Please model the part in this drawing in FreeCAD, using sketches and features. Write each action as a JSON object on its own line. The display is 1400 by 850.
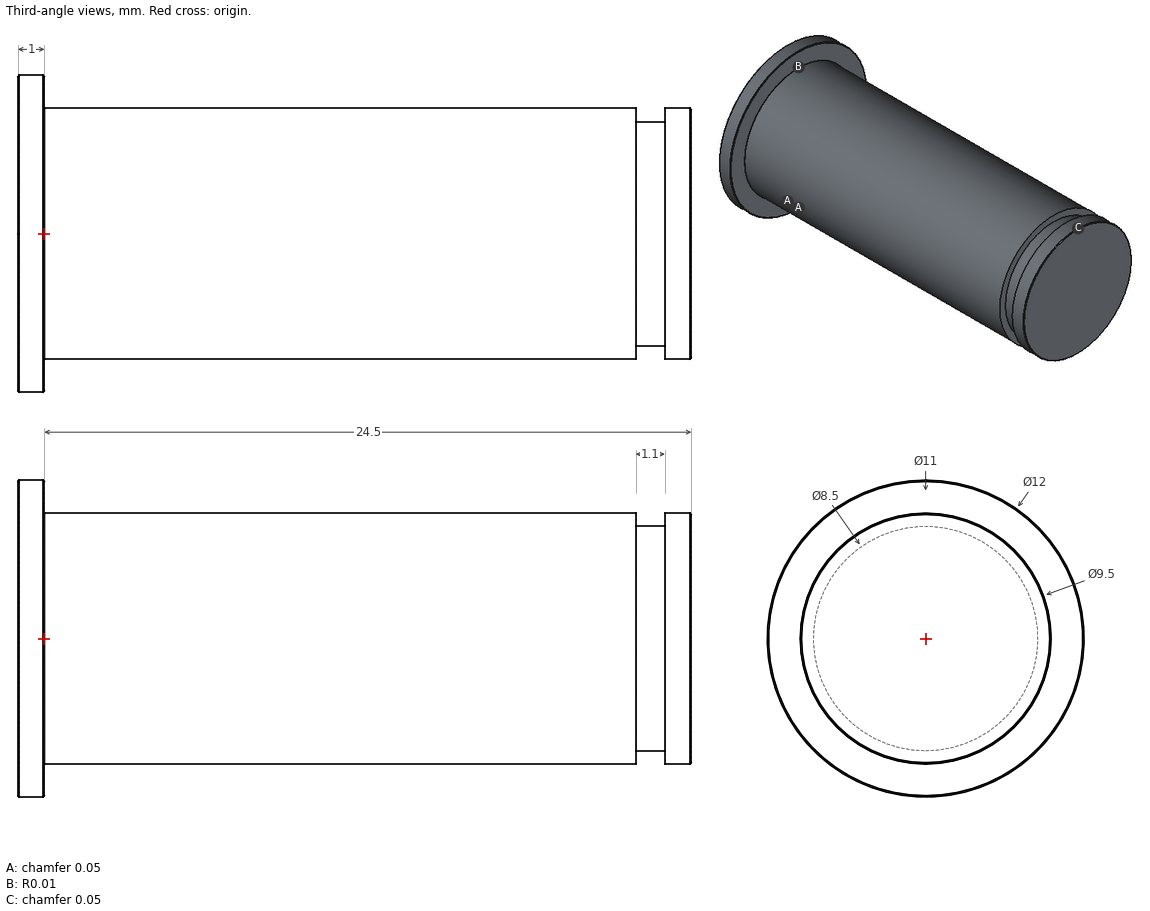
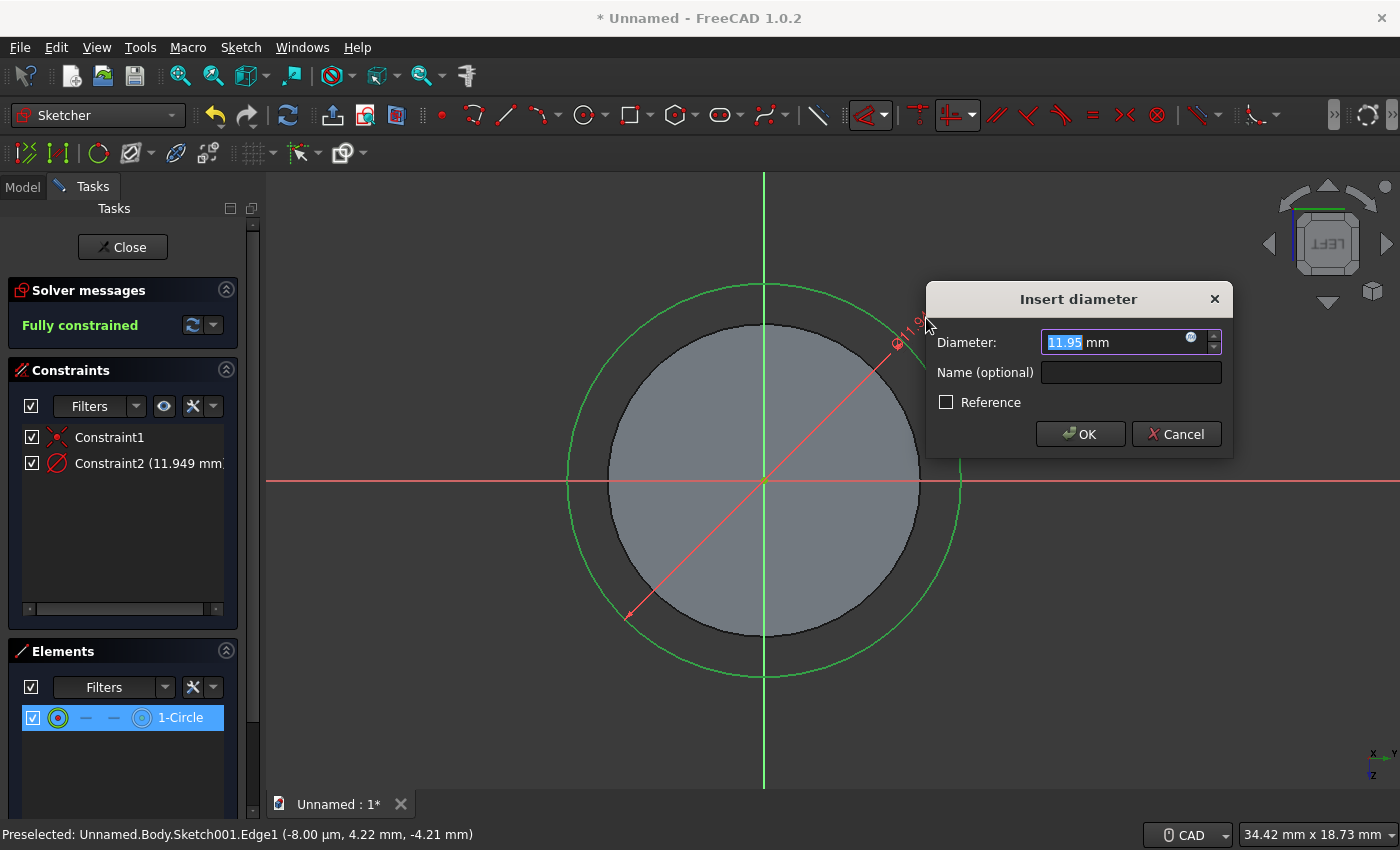
{"action": "type", "text": "12"}
{"action": "key", "text": "Return"}
{"action": "key", "text": "Escape"}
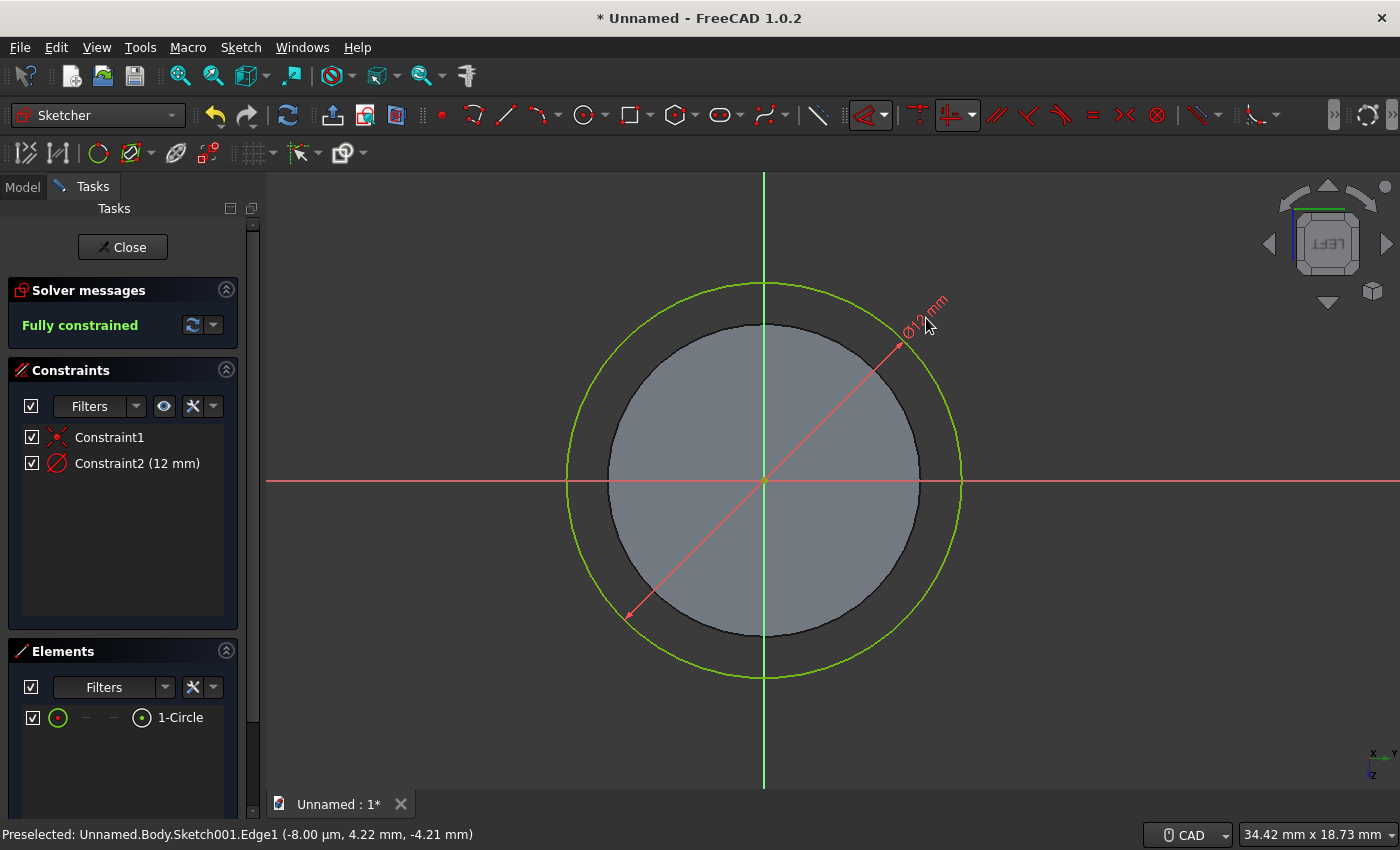
{"action": "left_click", "coordinate": [123, 247]}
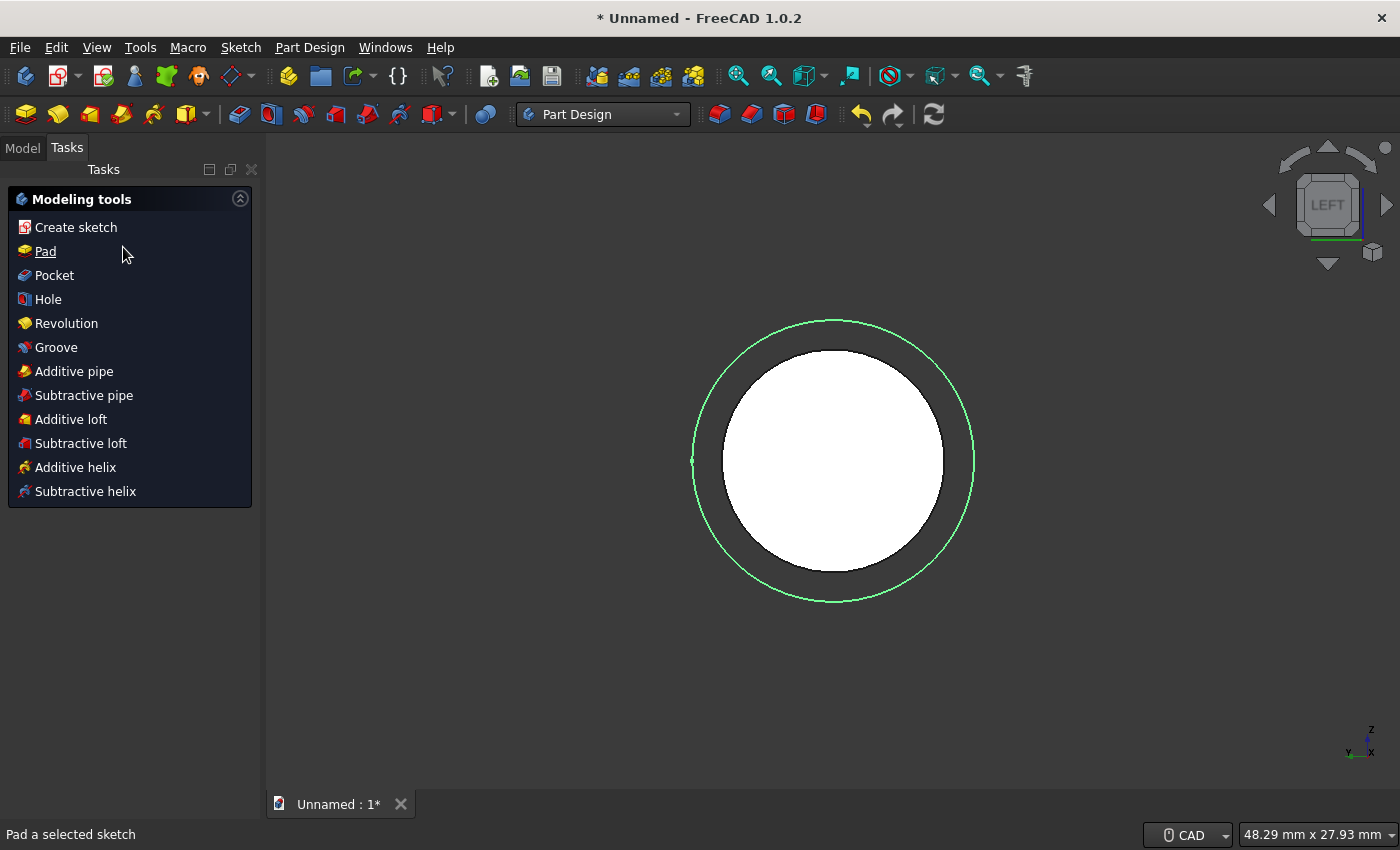
{"action": "left_click", "coordinate": [26, 114]}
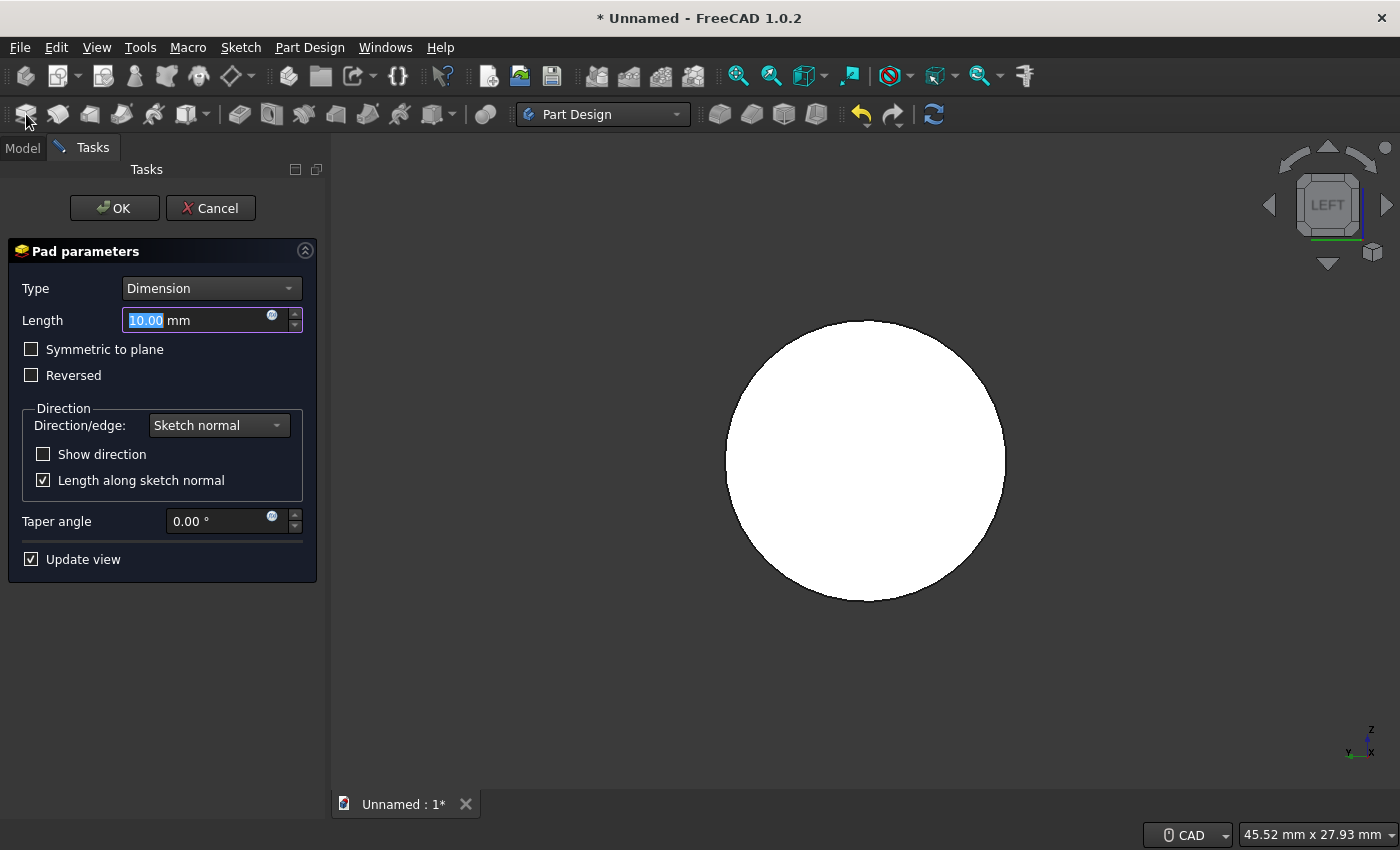
{"action": "type", "text": "1"}
{"action": "key", "text": "Tab"}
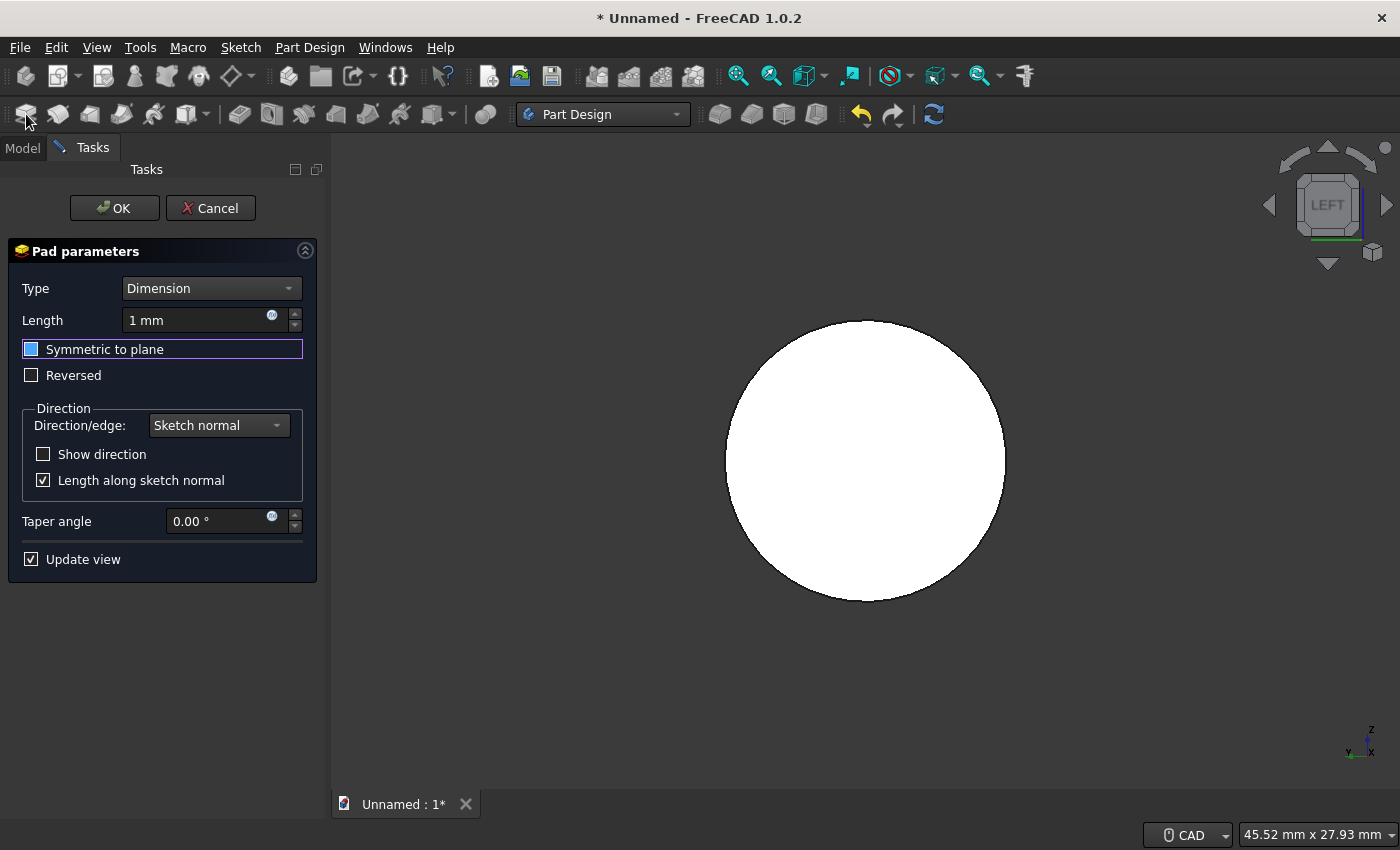
{"action": "left_click", "coordinate": [115, 208]}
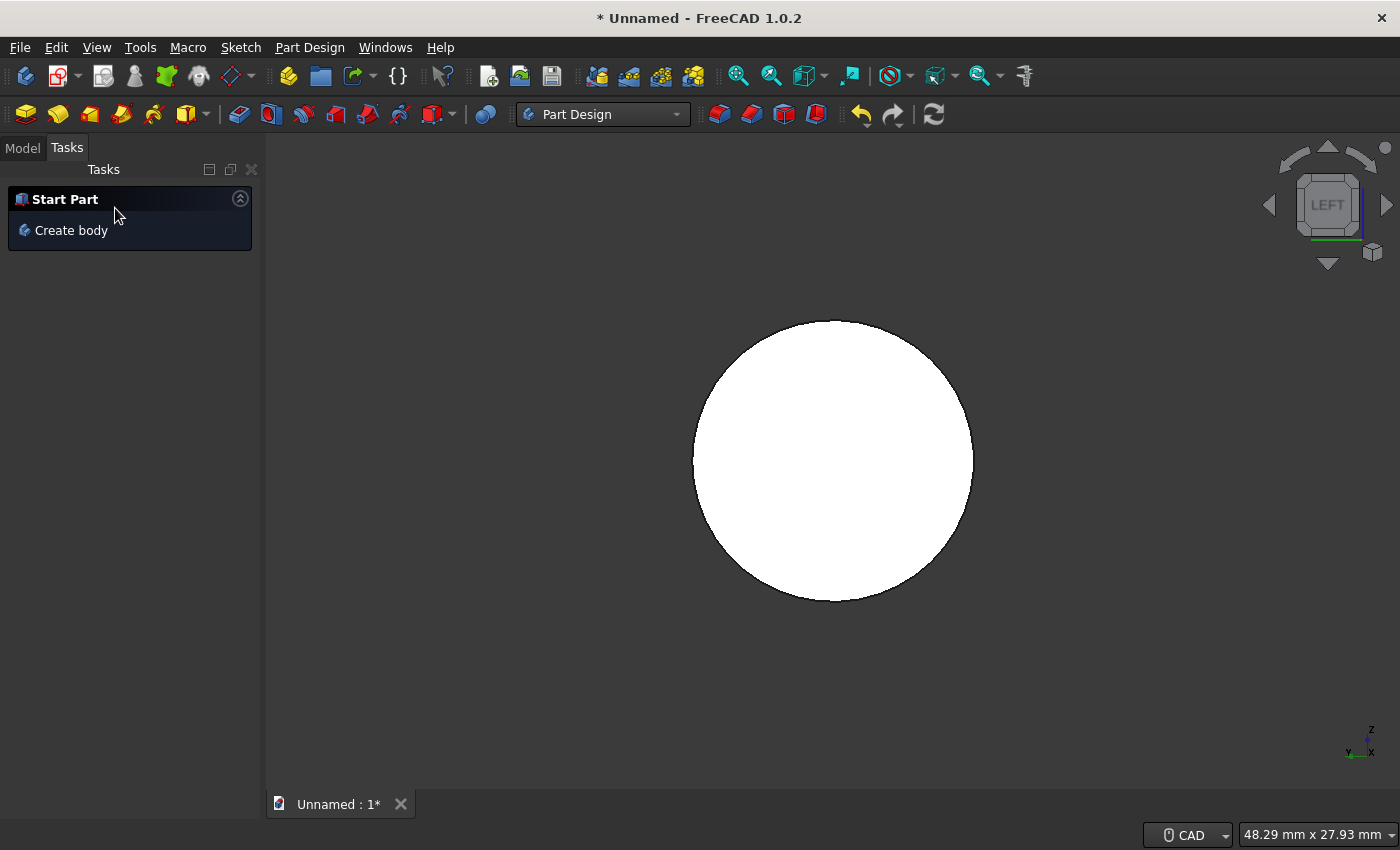
{"action": "key", "text": "v f"}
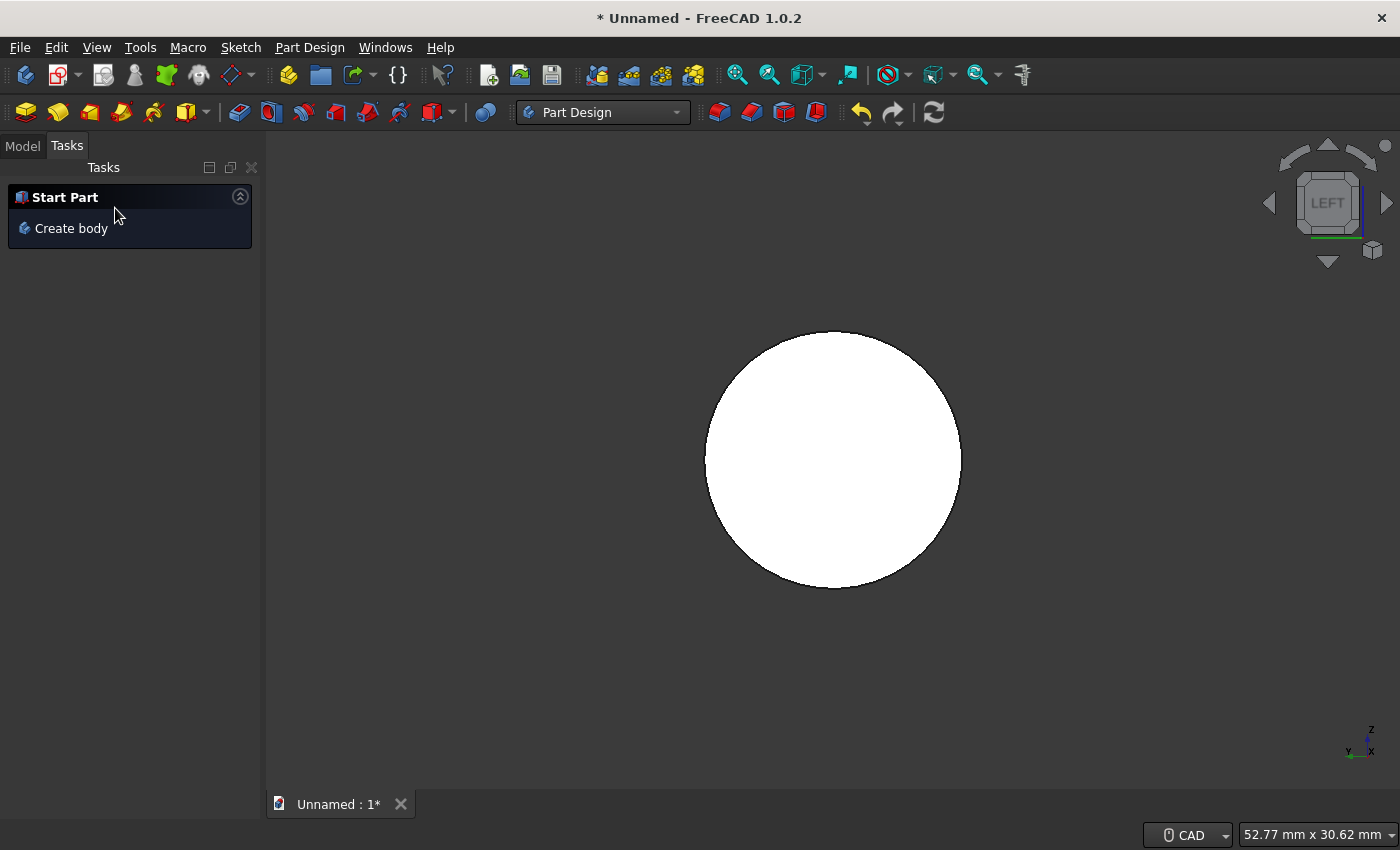
{"action": "left_click", "coordinate": [962, 459]}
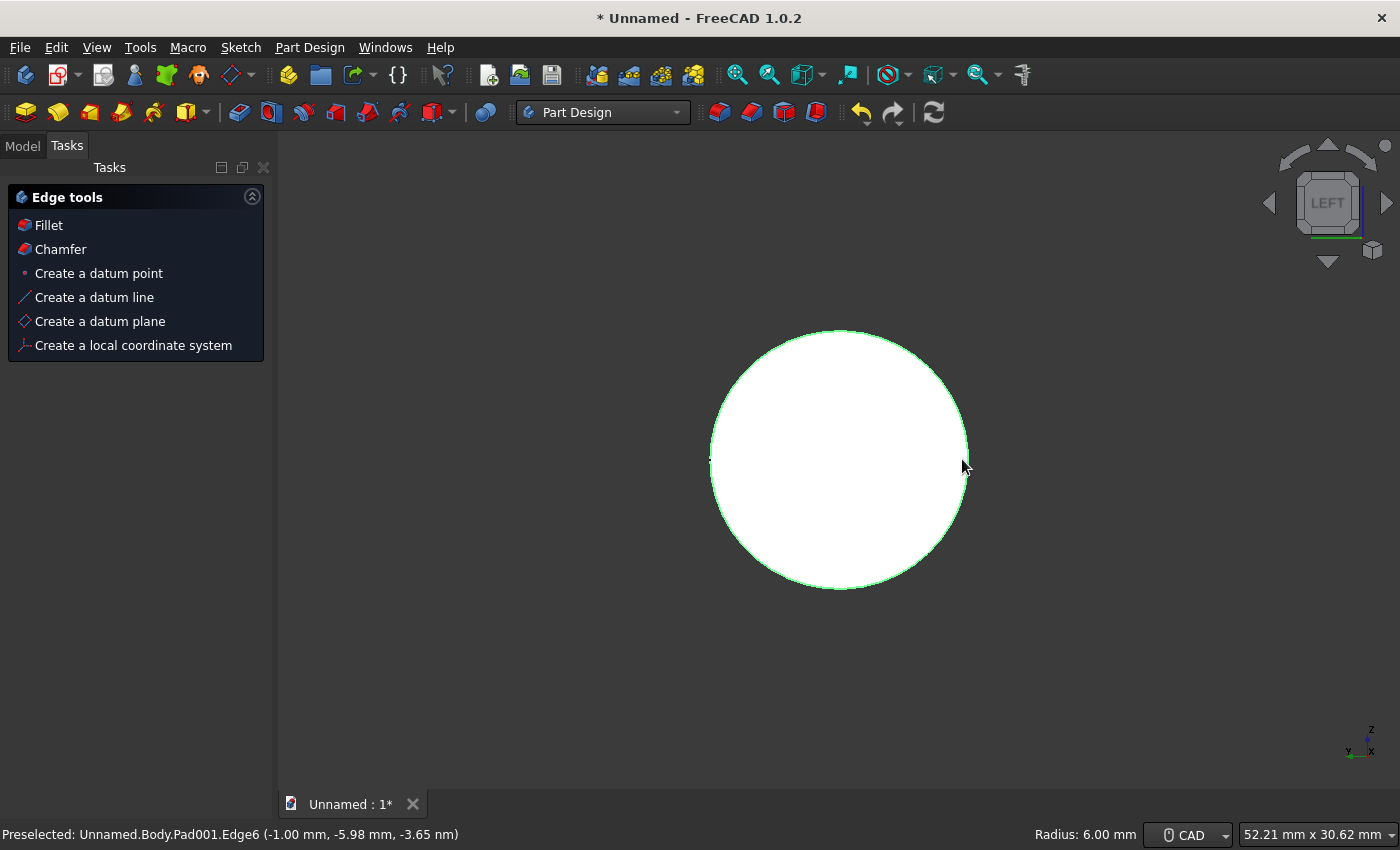
{"action": "key", "text": "0"}